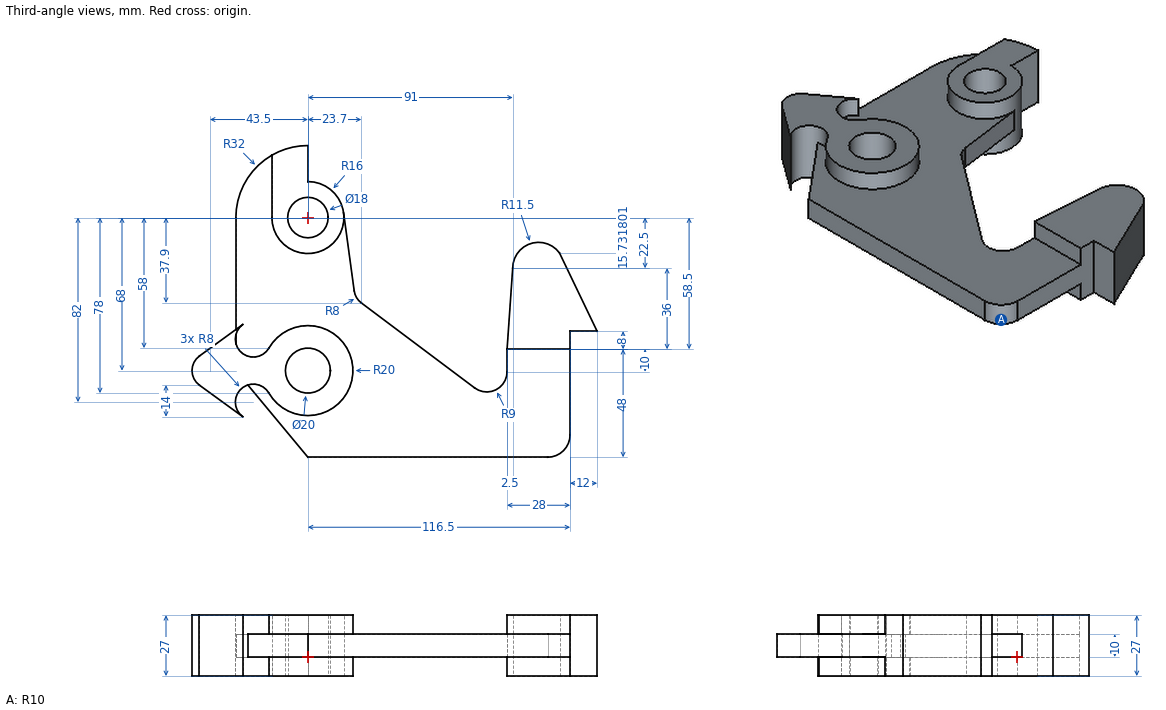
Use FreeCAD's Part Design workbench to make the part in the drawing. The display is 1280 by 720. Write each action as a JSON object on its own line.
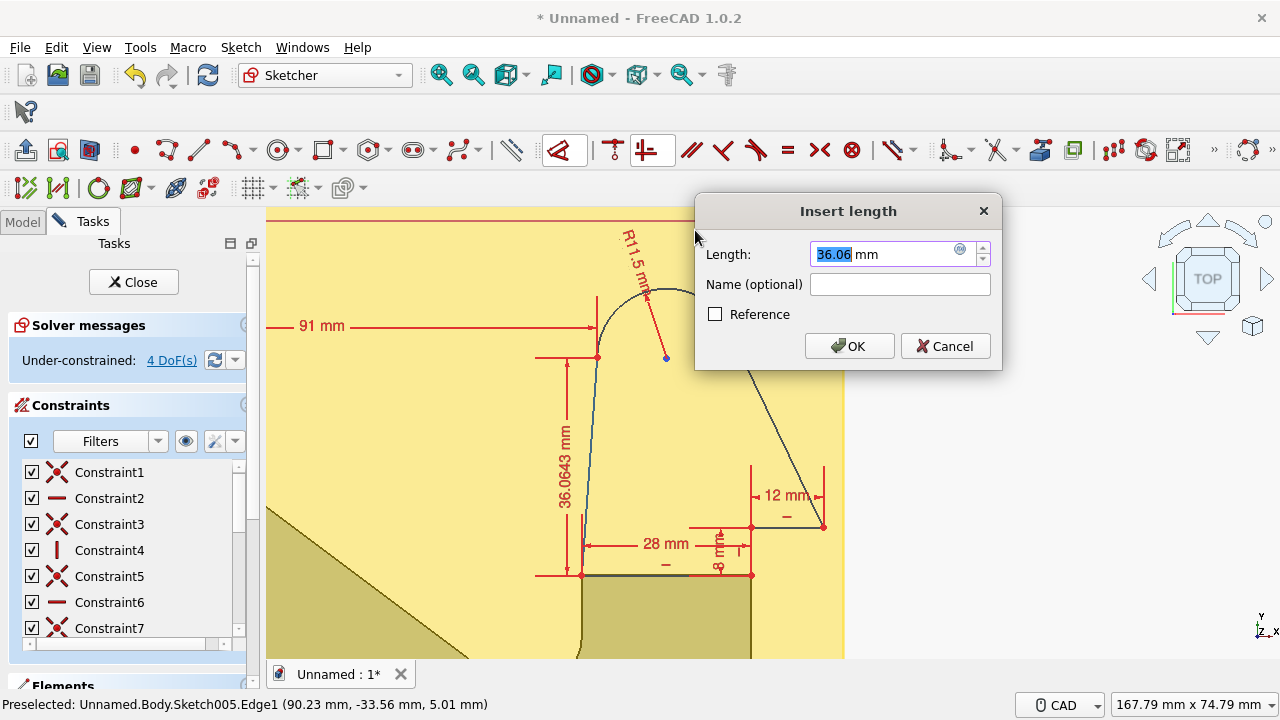
{"action": "type", "text": "36"}
{"action": "key", "text": "Return"}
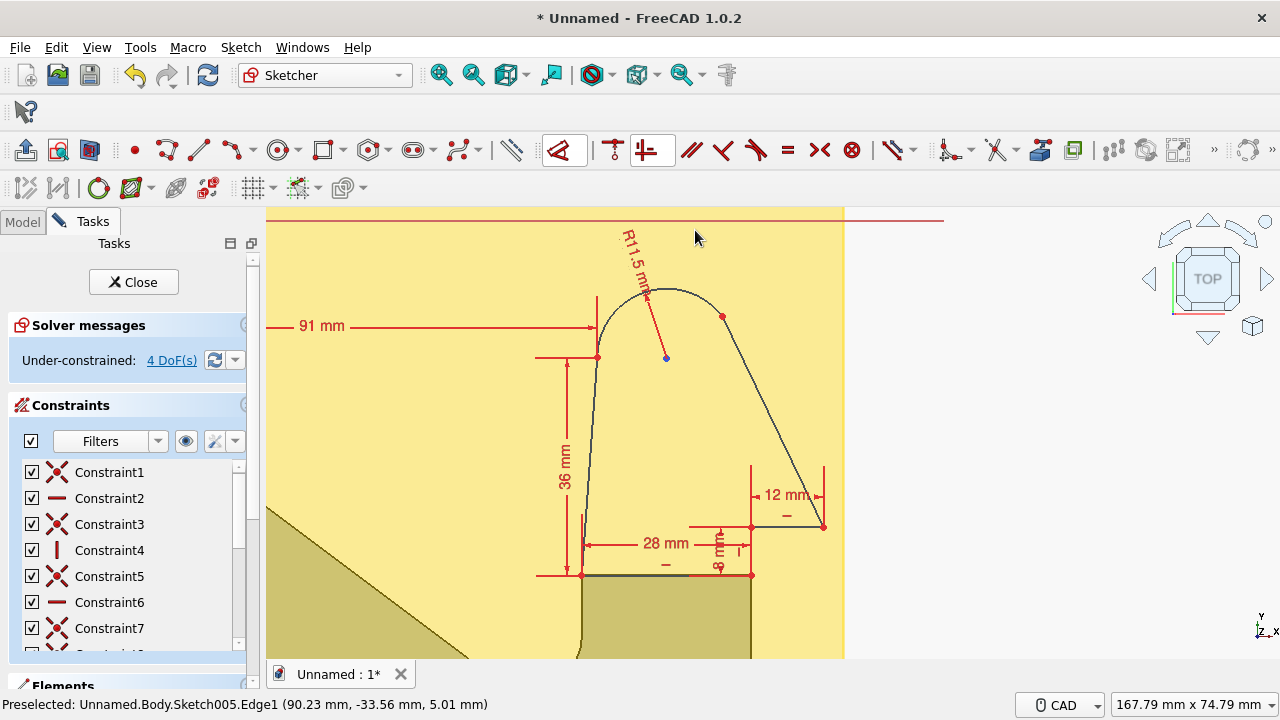
{"action": "scroll", "coordinate": [593, 423], "scroll_direction": "up", "scroll_amount": 5}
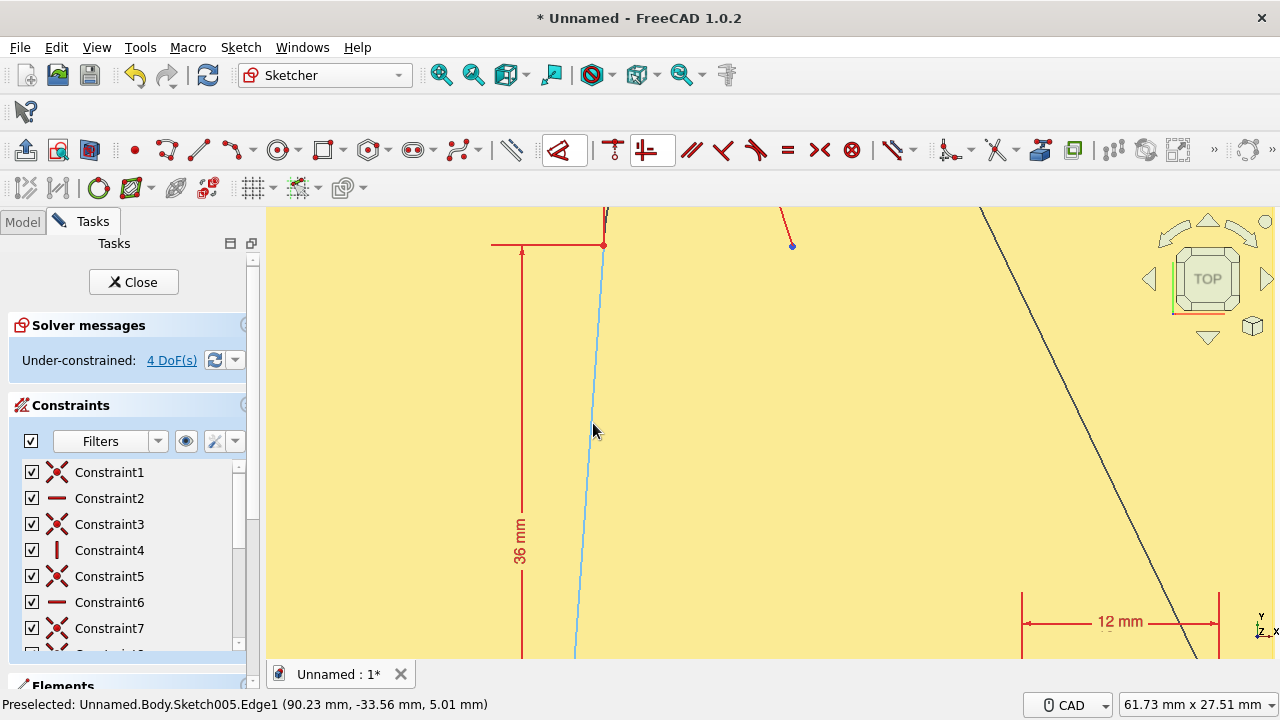
{"action": "left_click", "coordinate": [591, 423]}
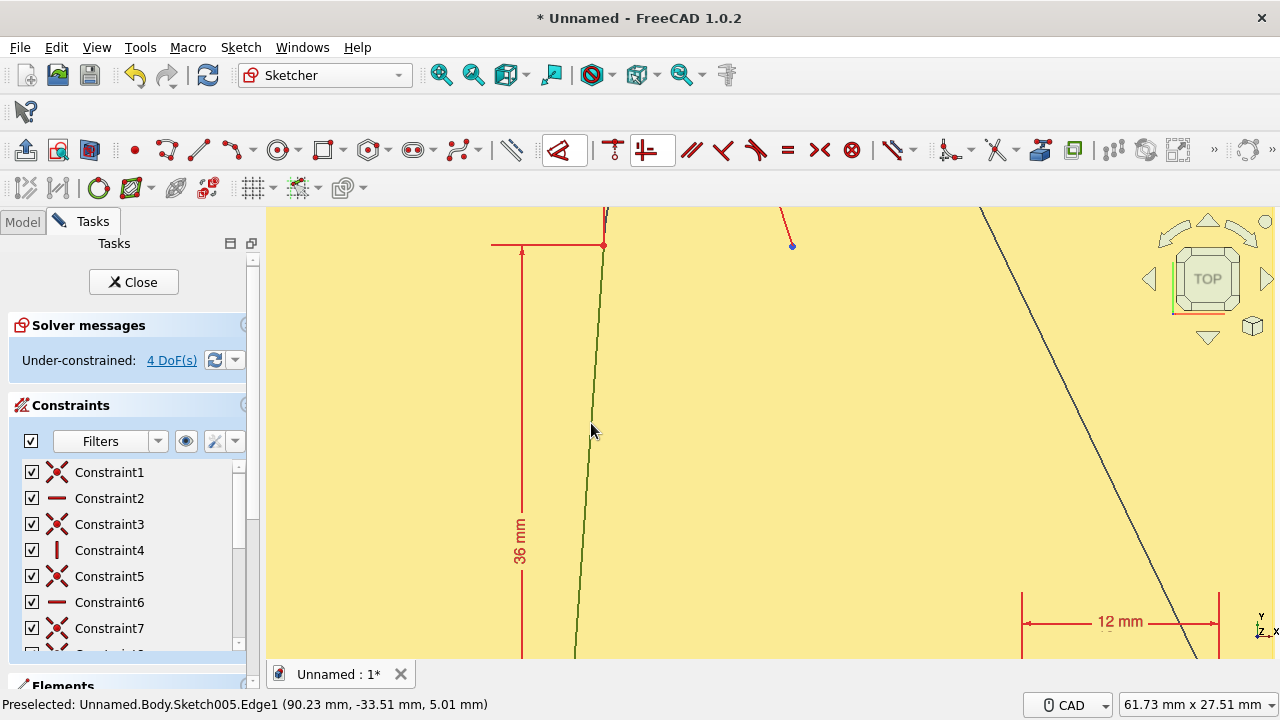
{"action": "key", "text": "l"}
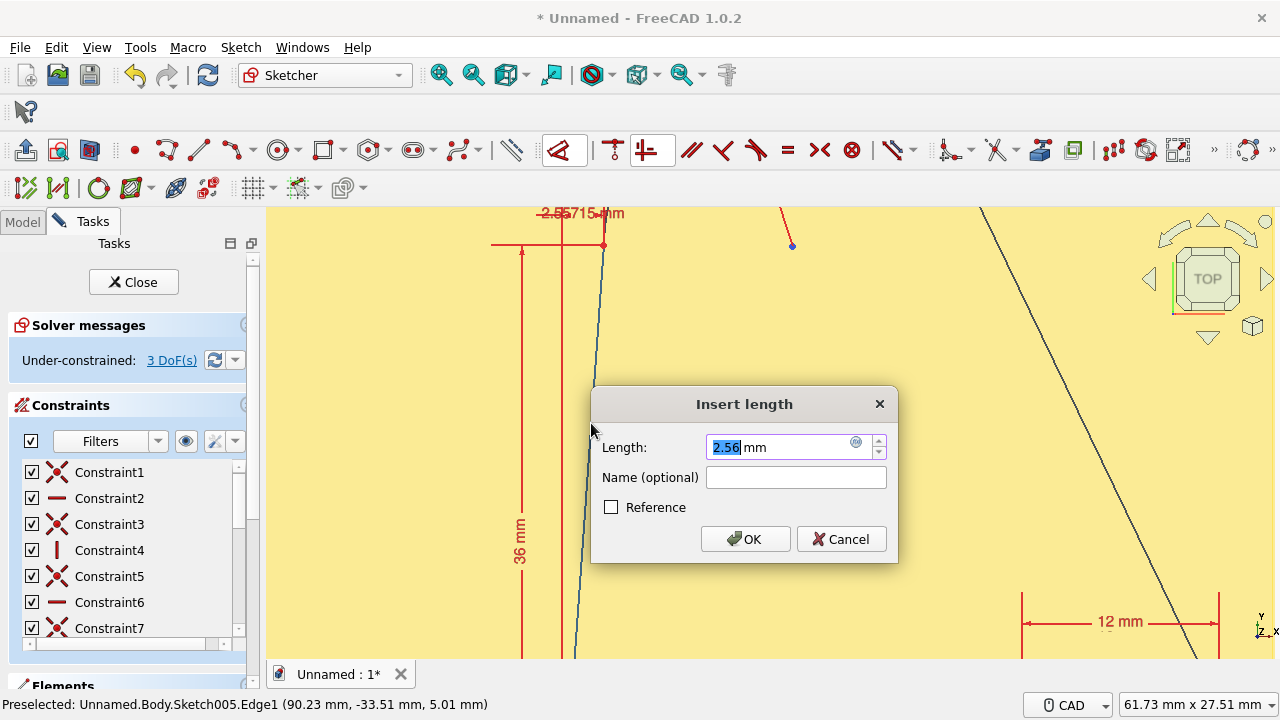
{"action": "type", "text": "2.5"}
{"action": "key", "text": "Return"}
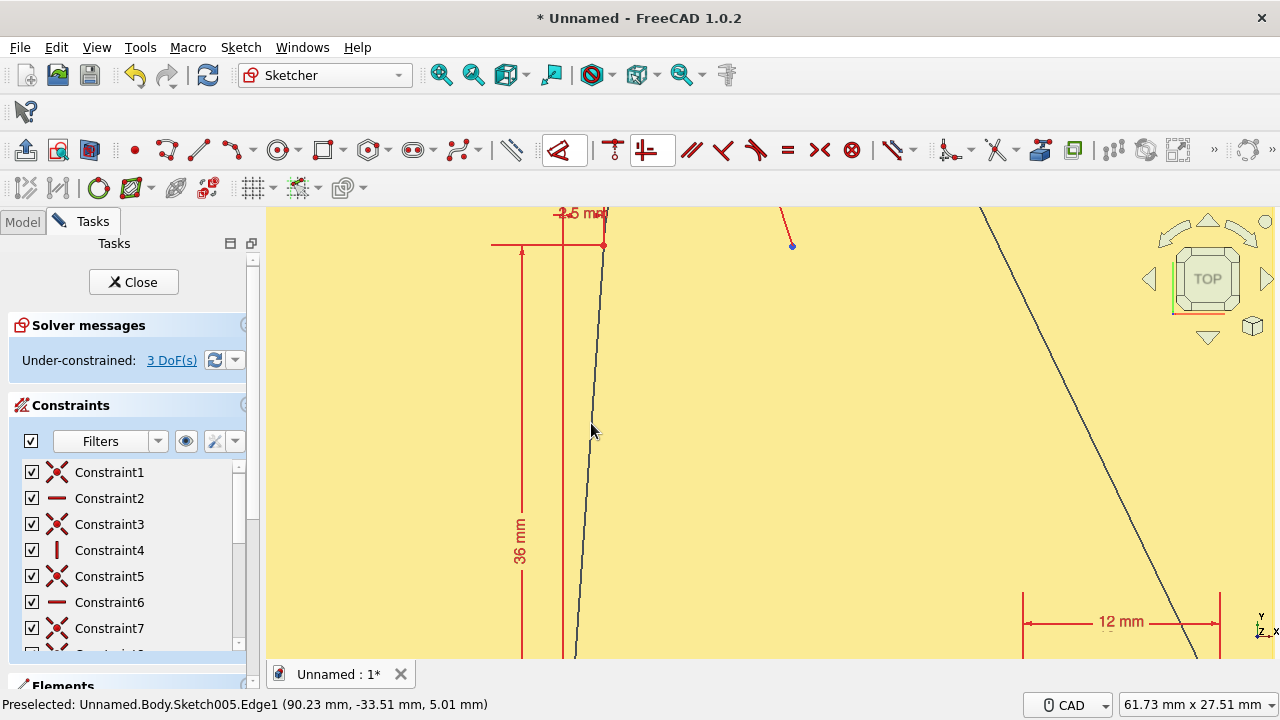
{"action": "left_click", "coordinate": [604, 245]}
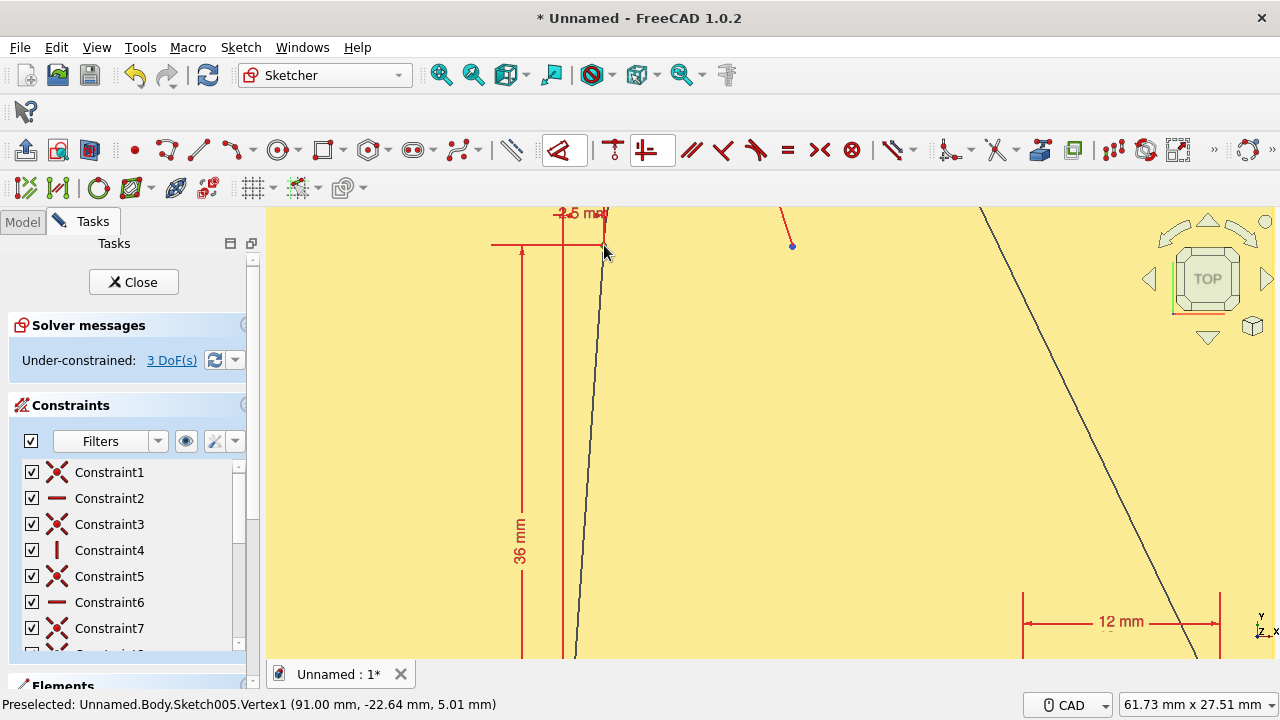
{"action": "left_click", "coordinate": [582, 150]}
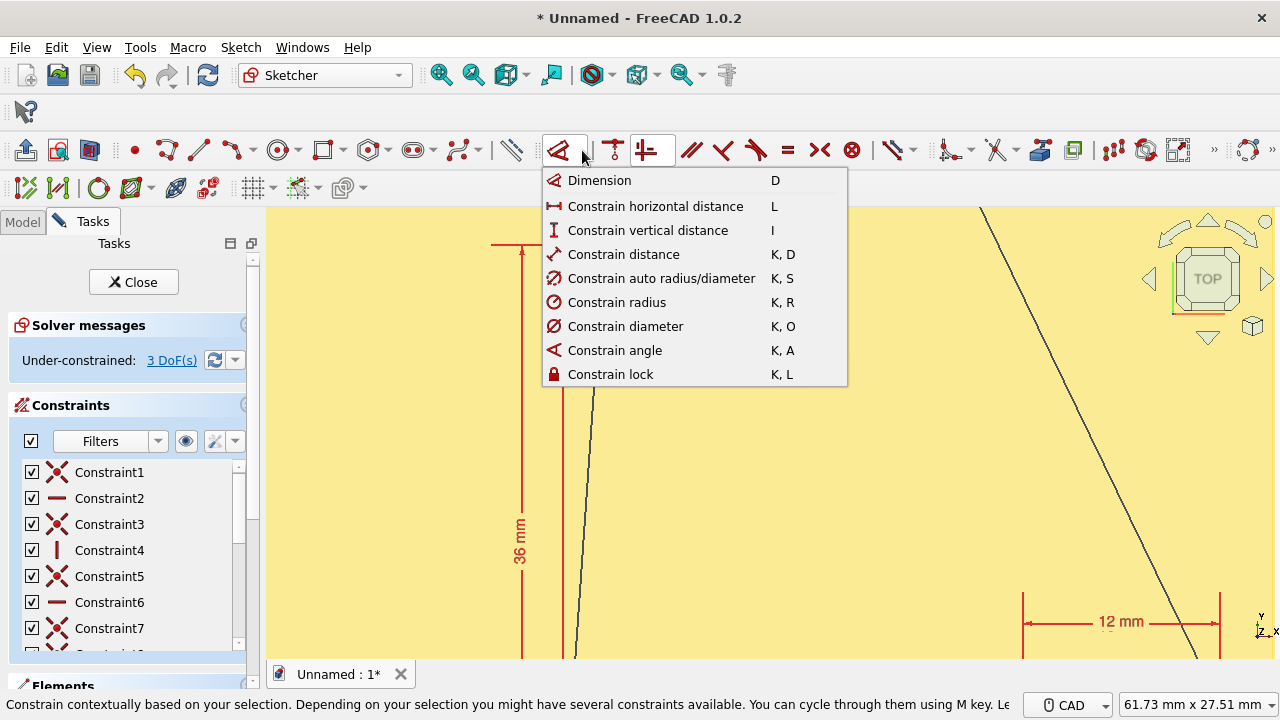
{"action": "left_click", "coordinate": [695, 230]}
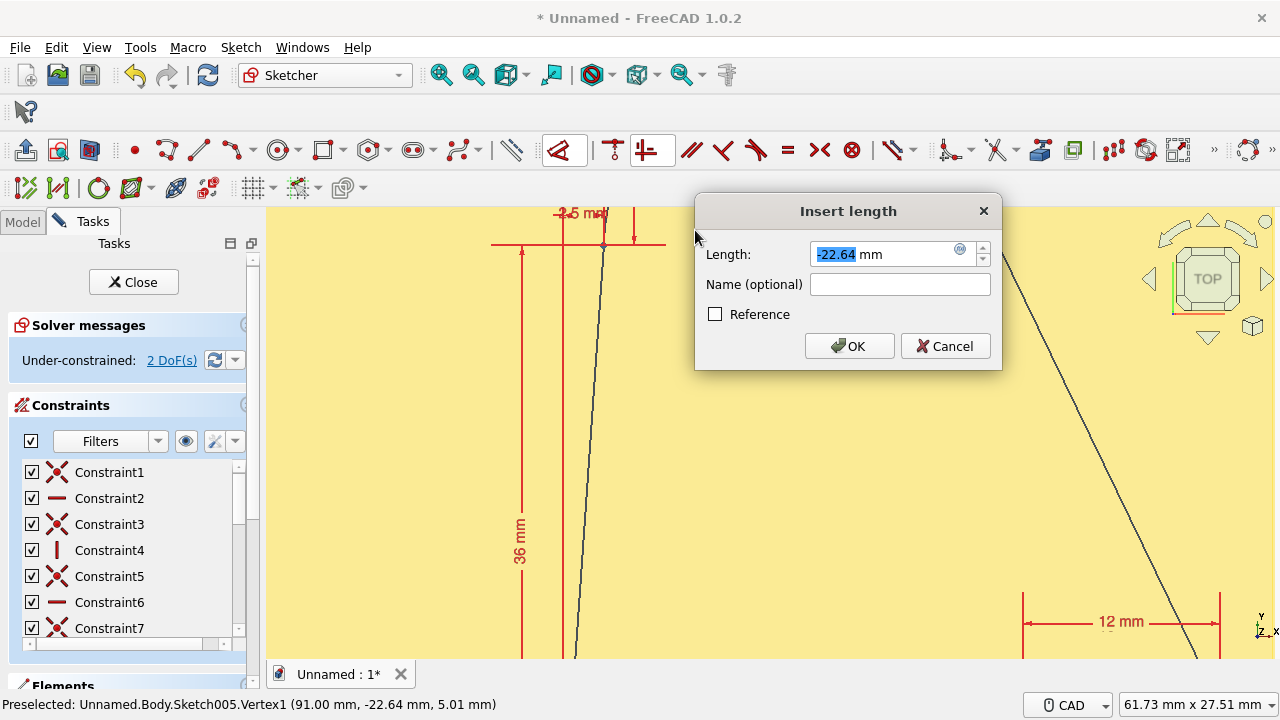
{"action": "type", "text": "-22.5"}
{"action": "key", "text": "Return"}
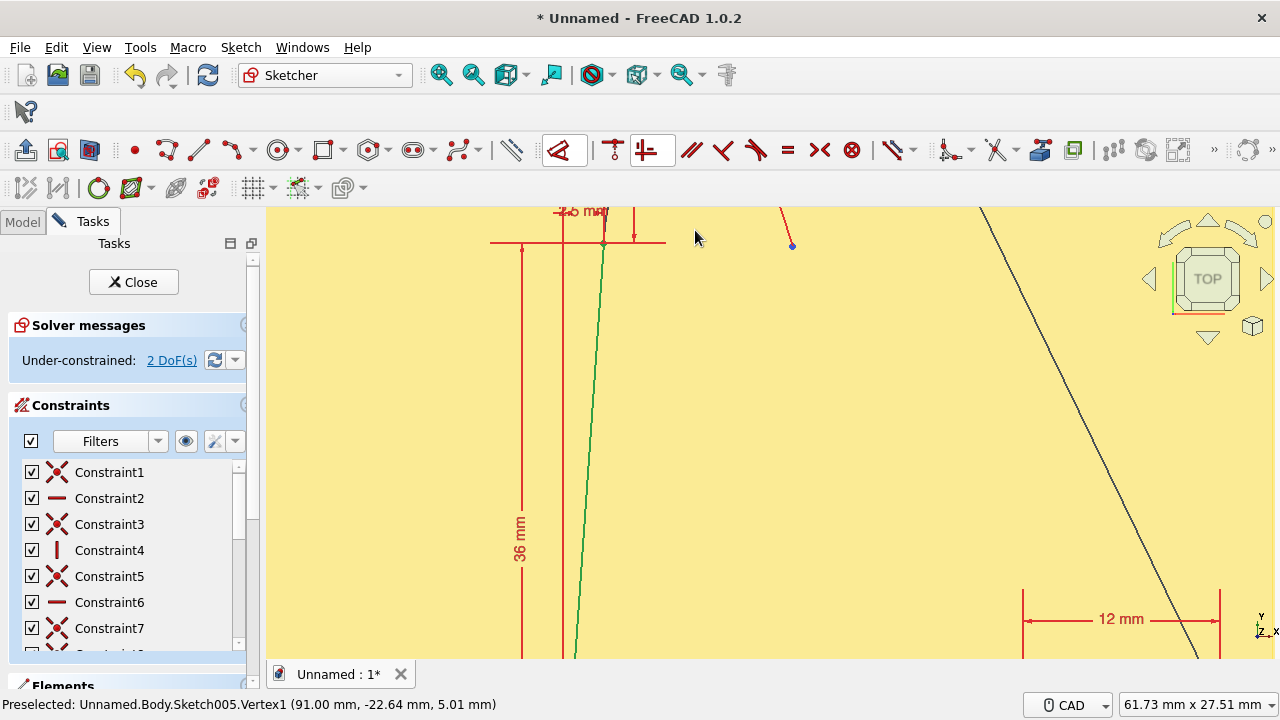
{"action": "left_click", "coordinate": [793, 246]}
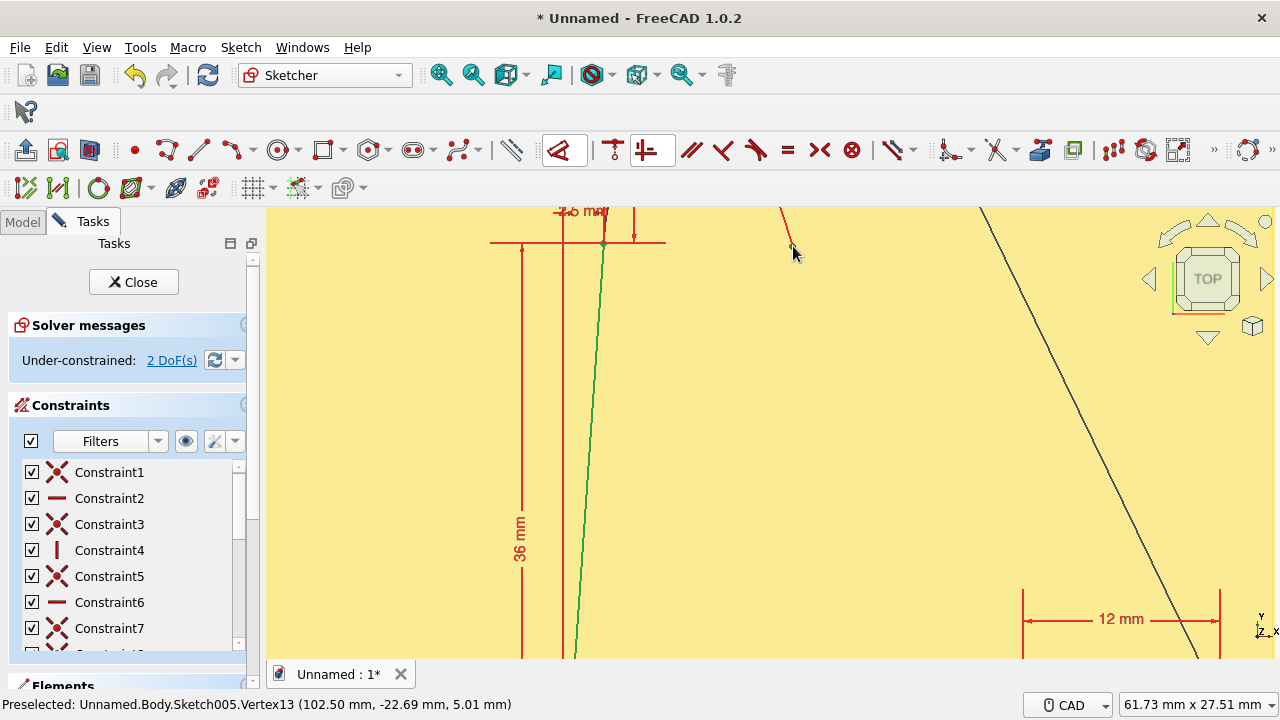
{"action": "key", "text": "i"}